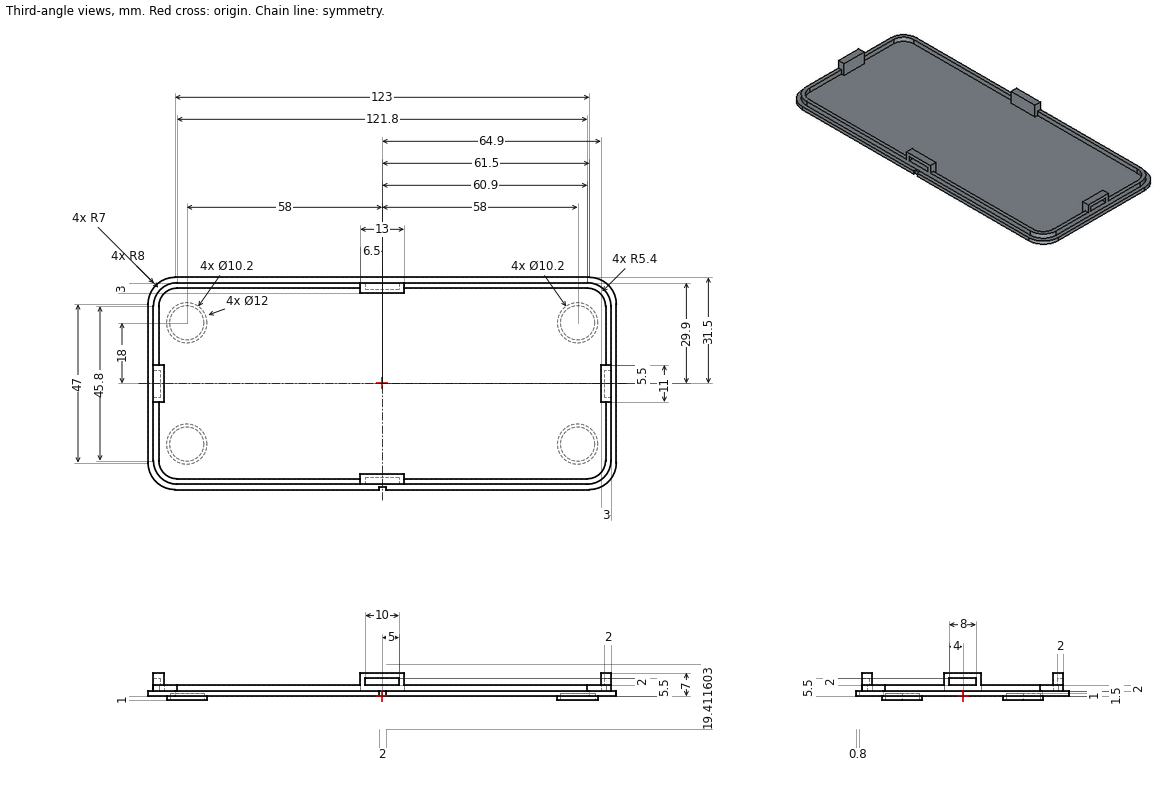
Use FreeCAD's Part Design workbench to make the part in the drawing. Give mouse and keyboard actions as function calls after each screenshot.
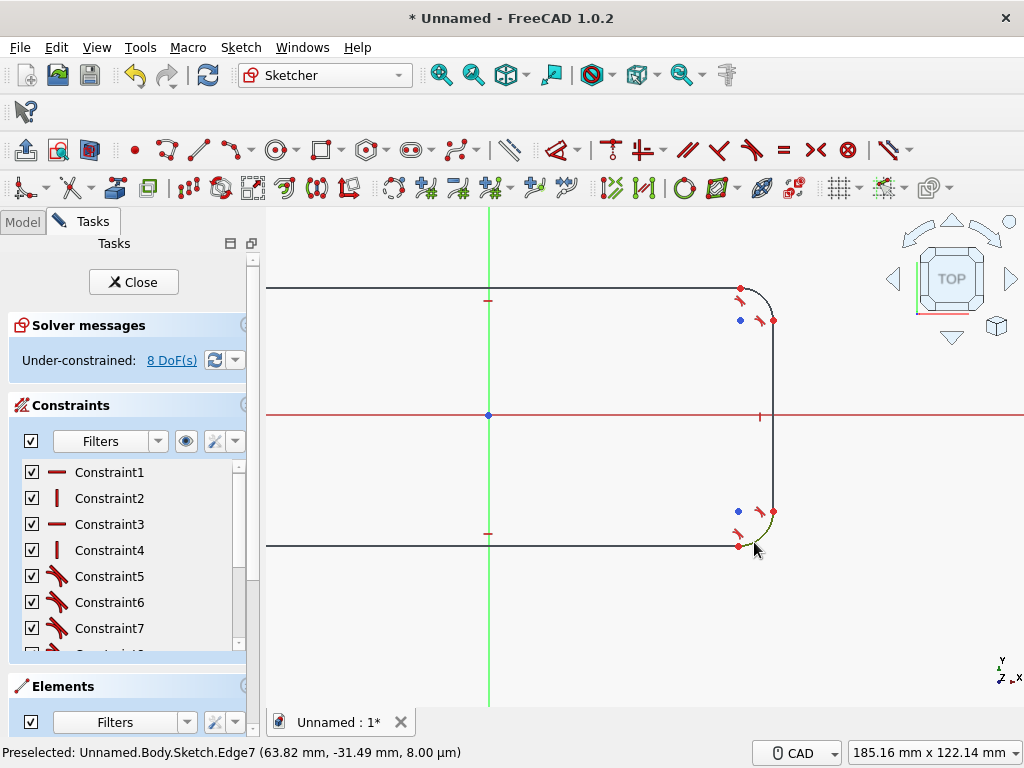
click(769, 306)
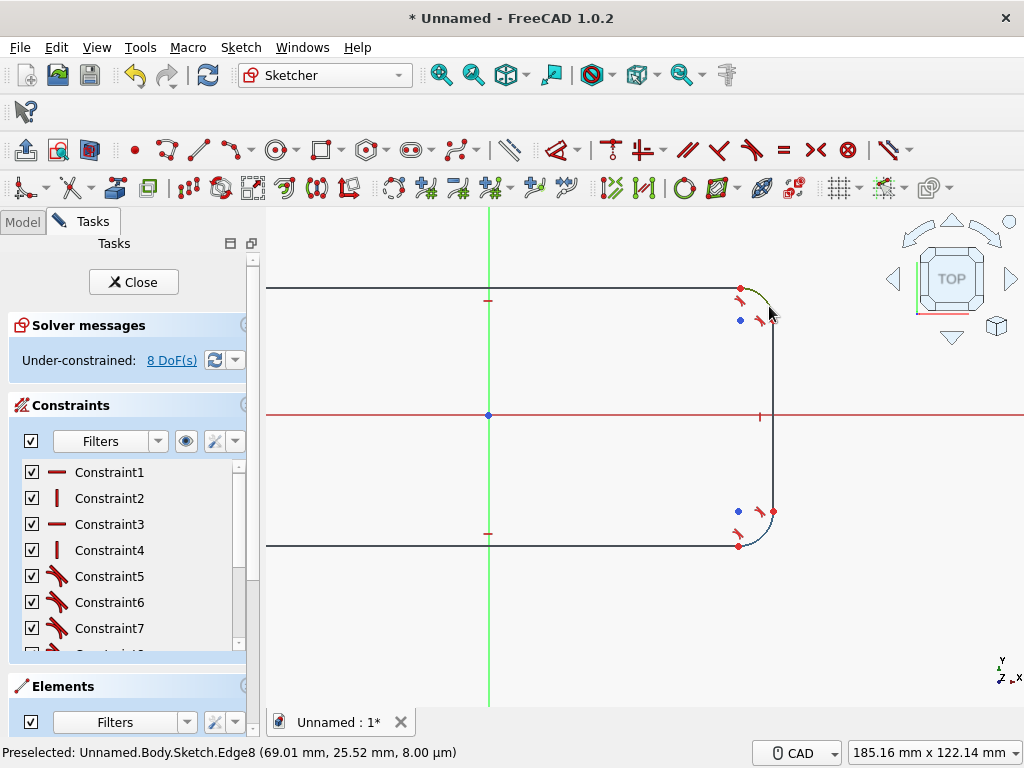
click(784, 150)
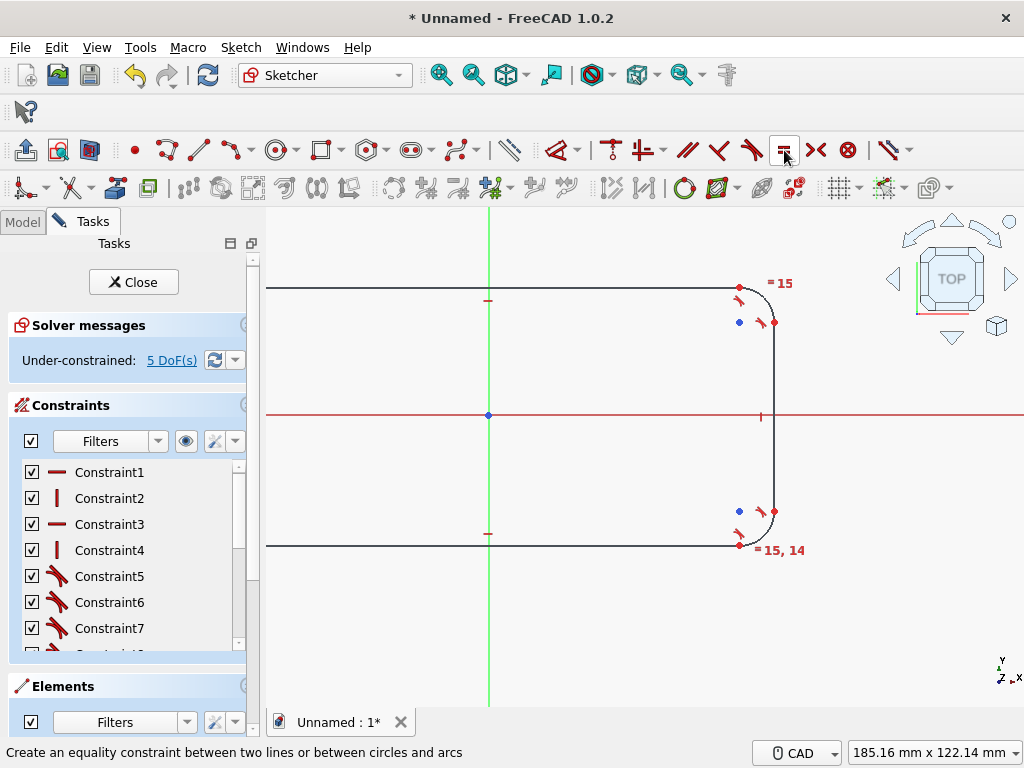
scroll(755, 542, down, 2)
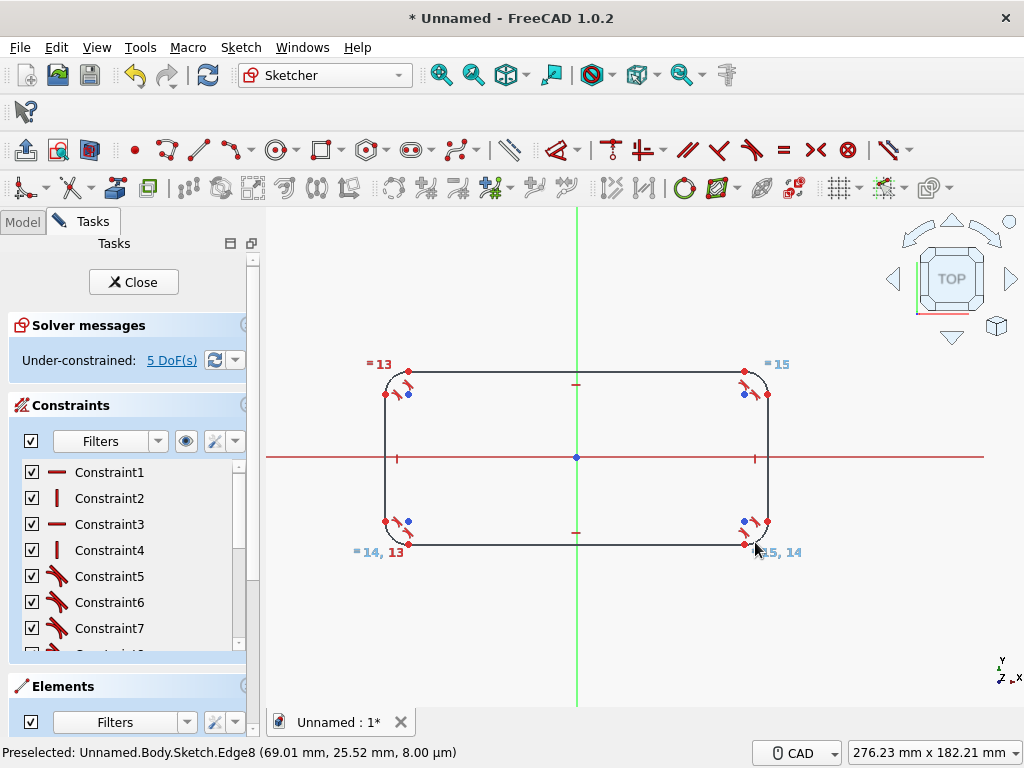
scroll(398, 374, up, 3)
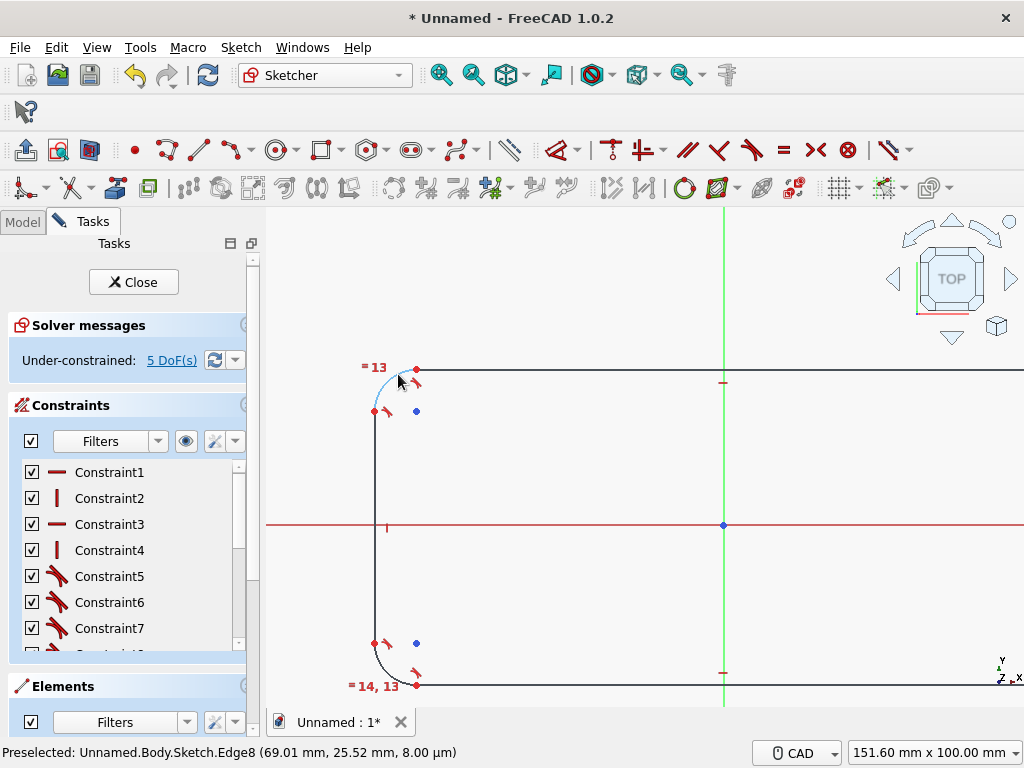
click(398, 374)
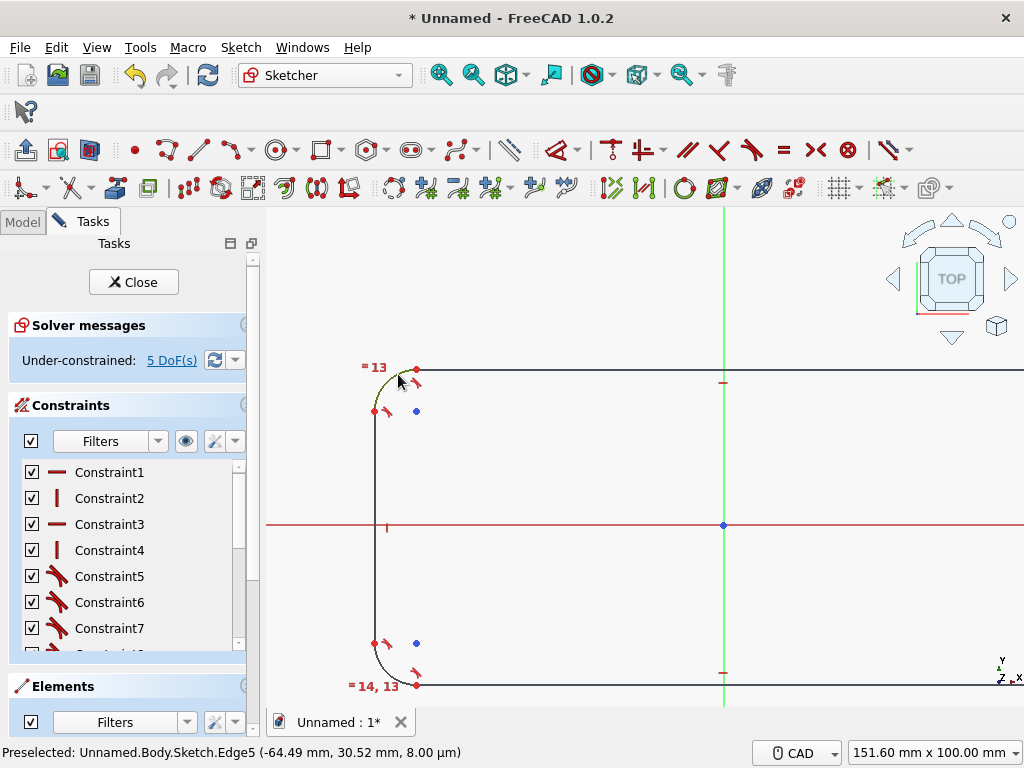
key(k)
key(r)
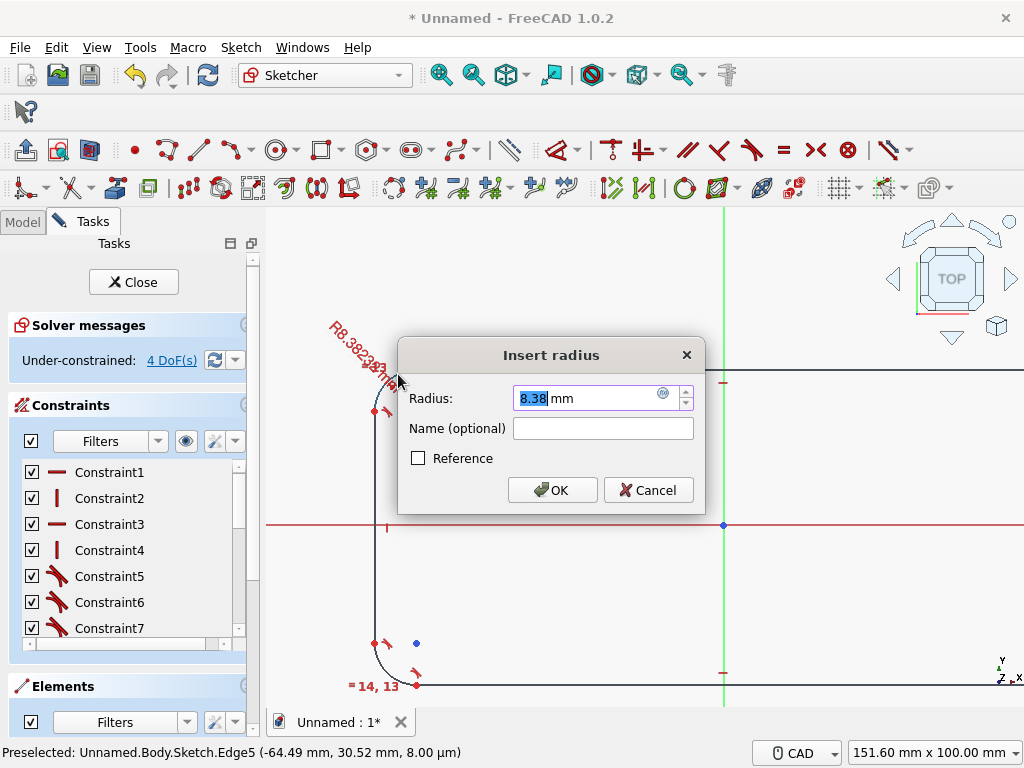
text(8)
key(Return)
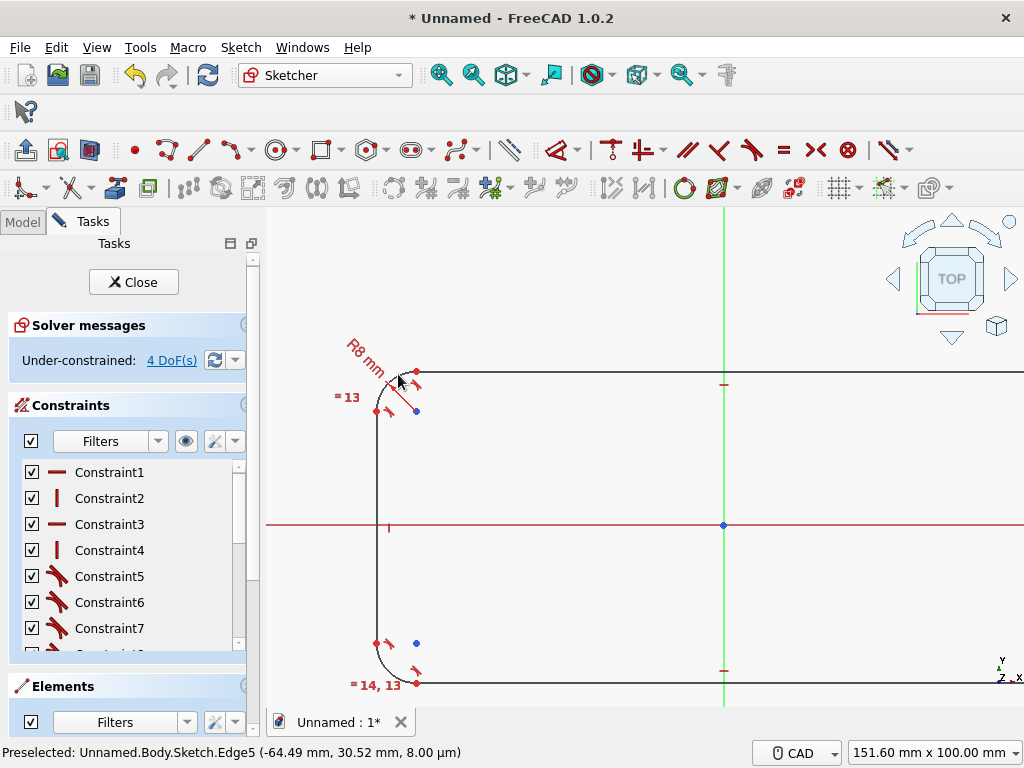
click(377, 481)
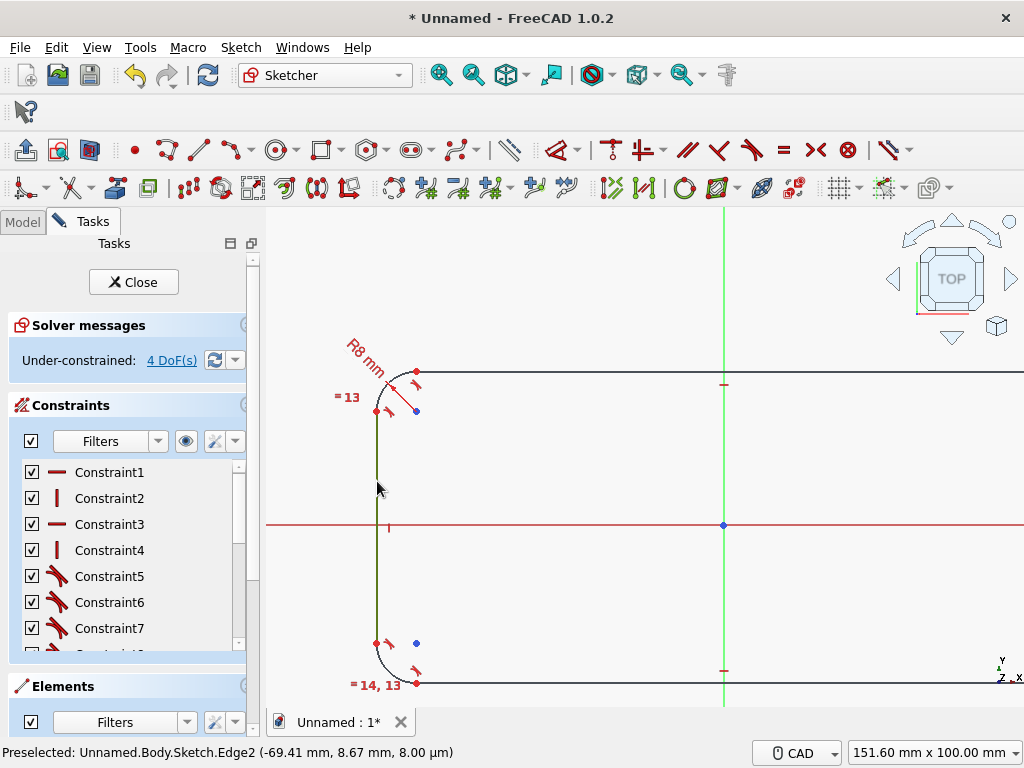
click(580, 150)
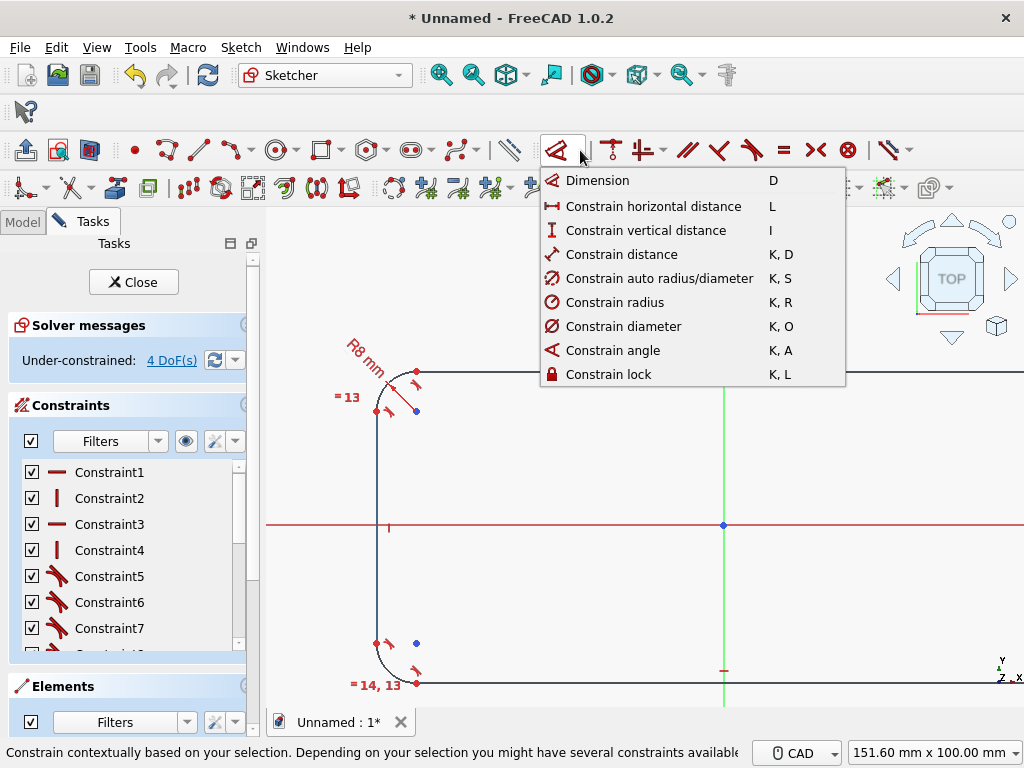
click(693, 230)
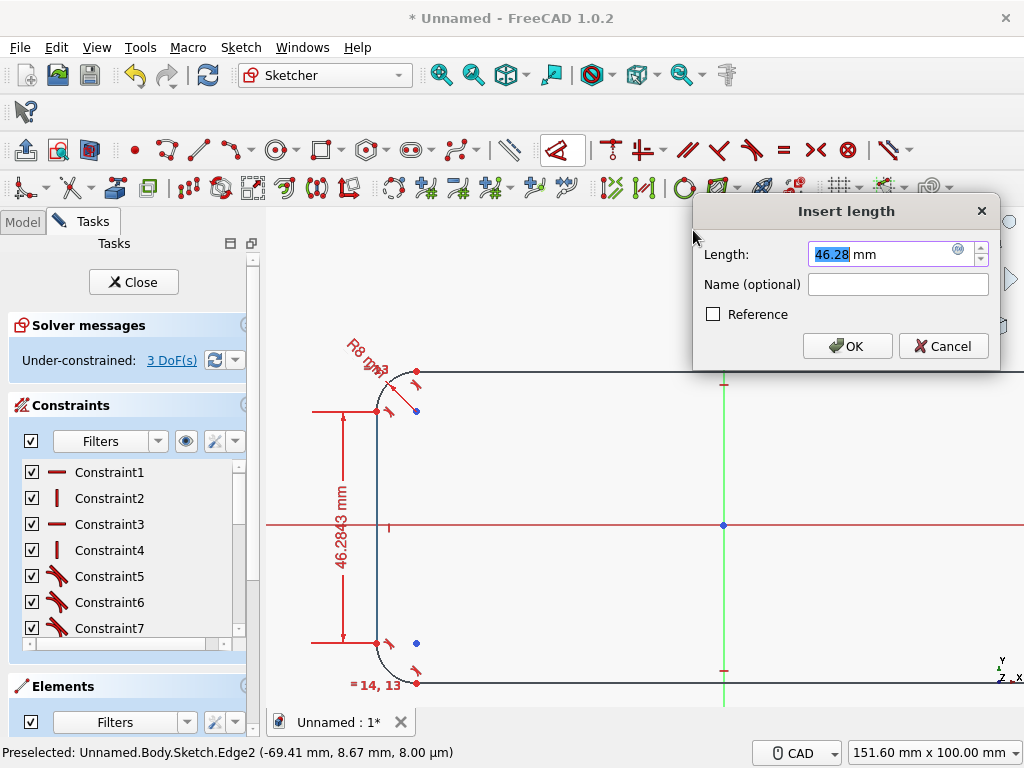
text(47)
key(Return)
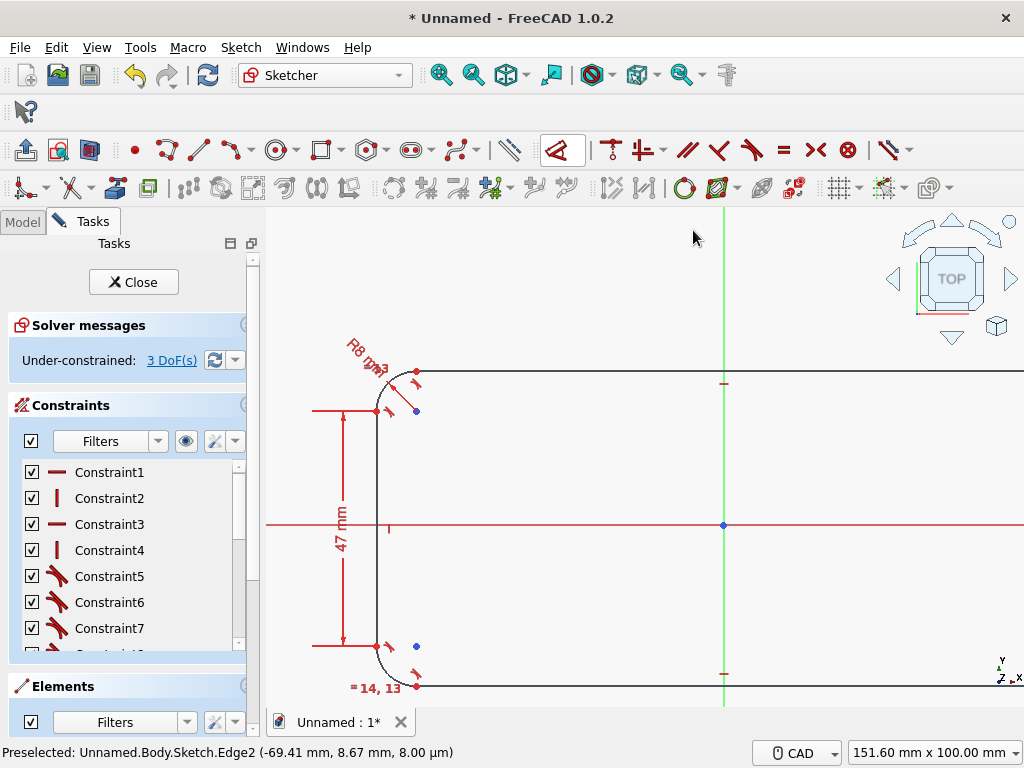
click(847, 371)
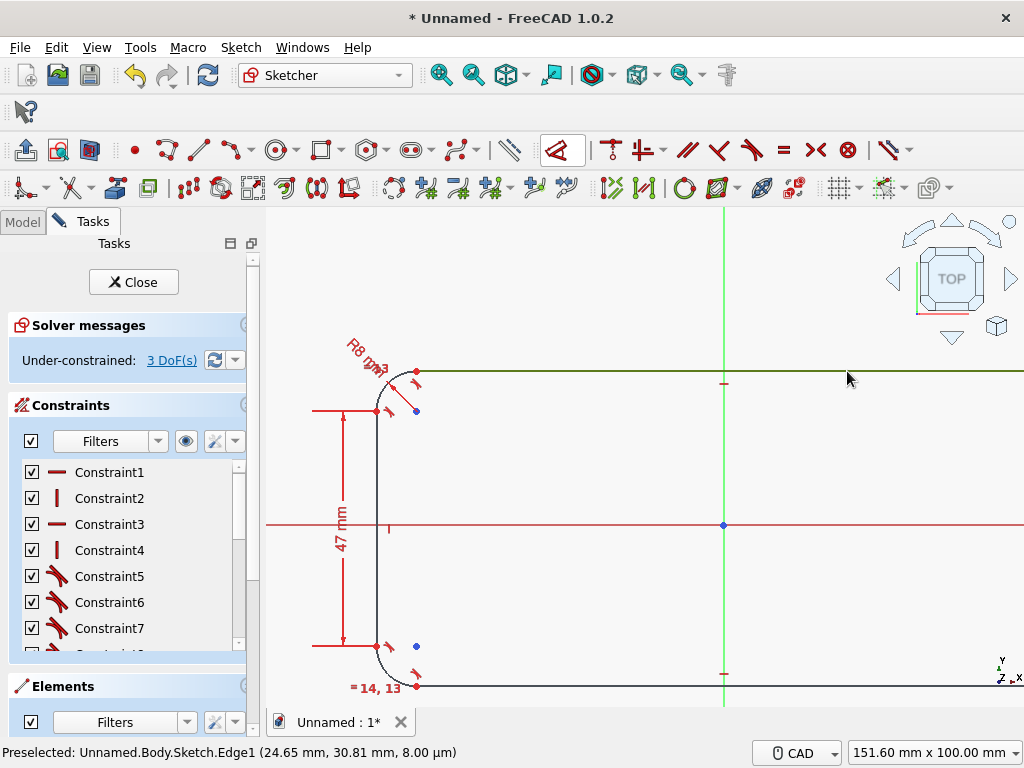
key(l)